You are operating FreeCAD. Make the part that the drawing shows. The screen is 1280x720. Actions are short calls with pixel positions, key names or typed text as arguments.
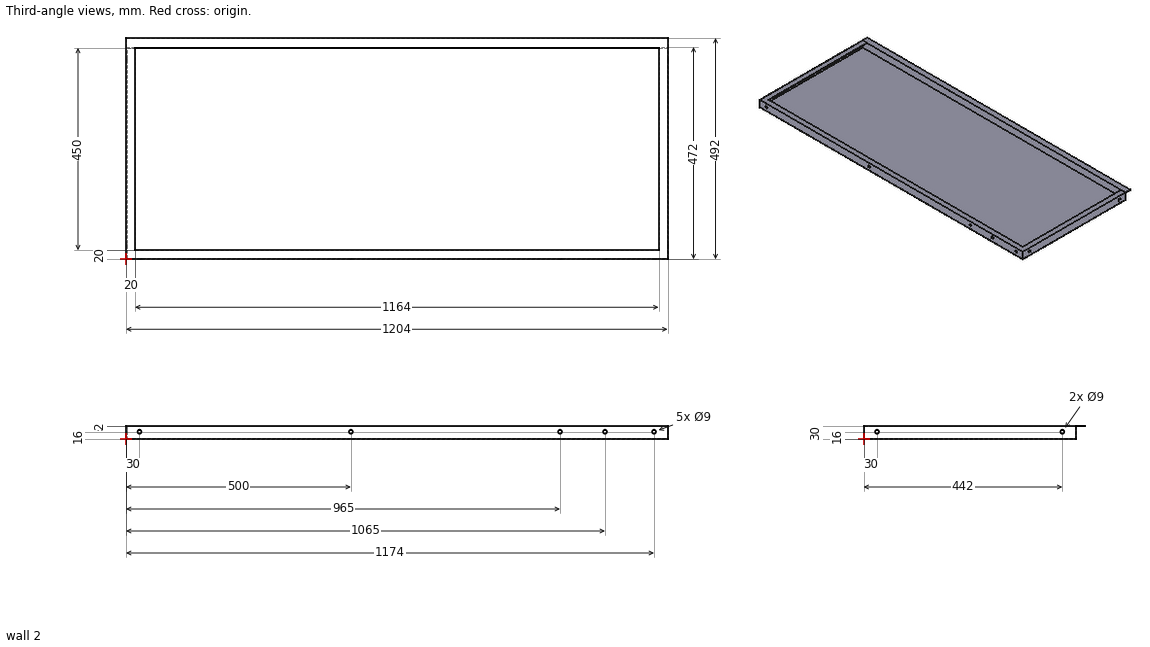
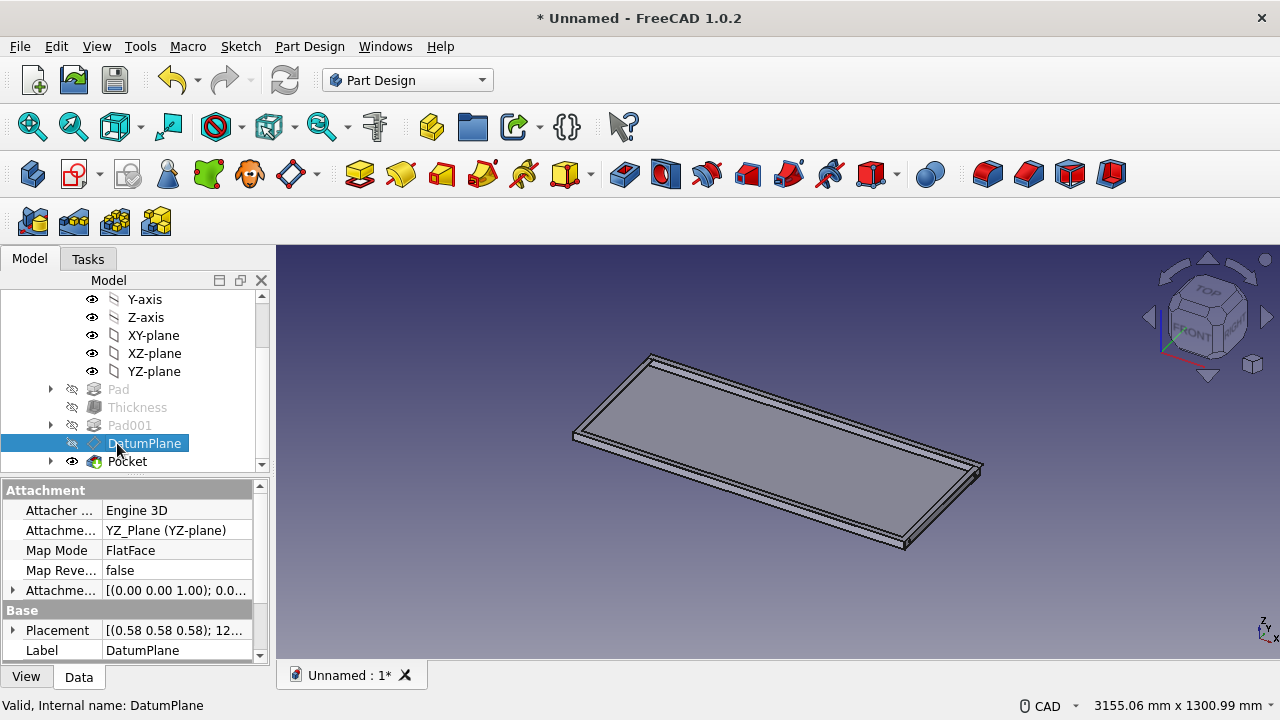
scroll(161, 385, down, 3)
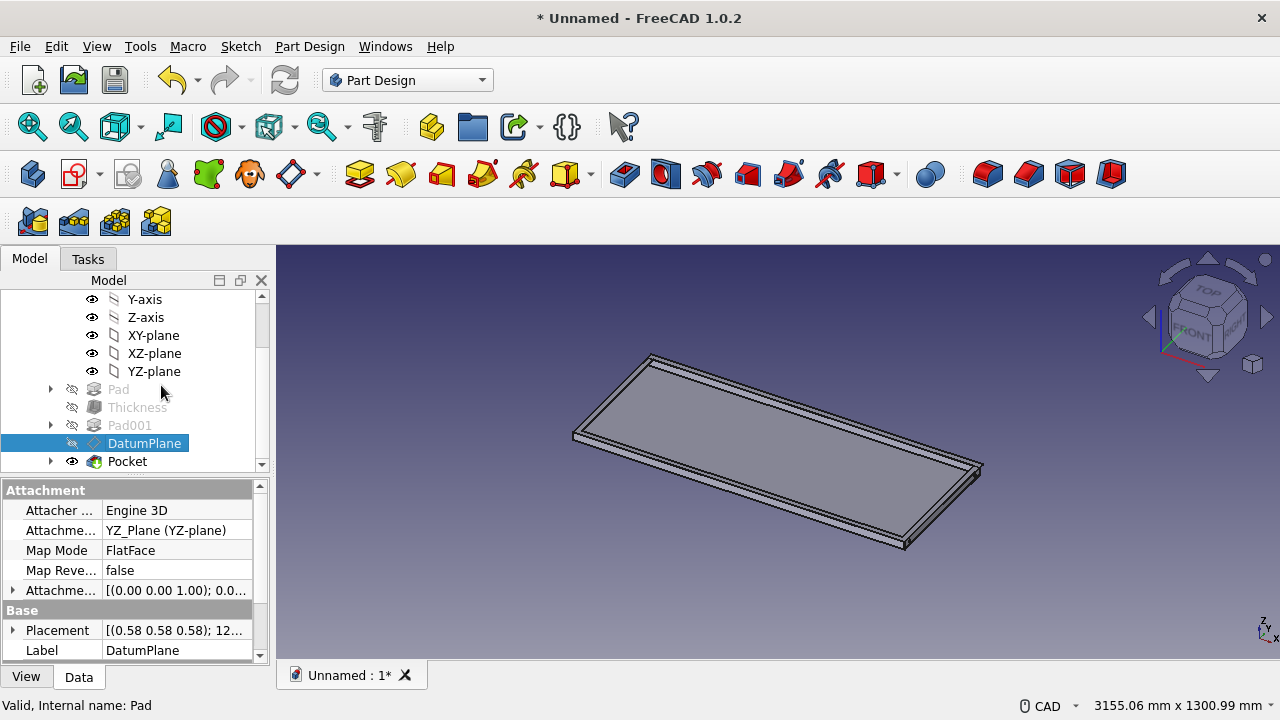
scroll(161, 385, up, 15)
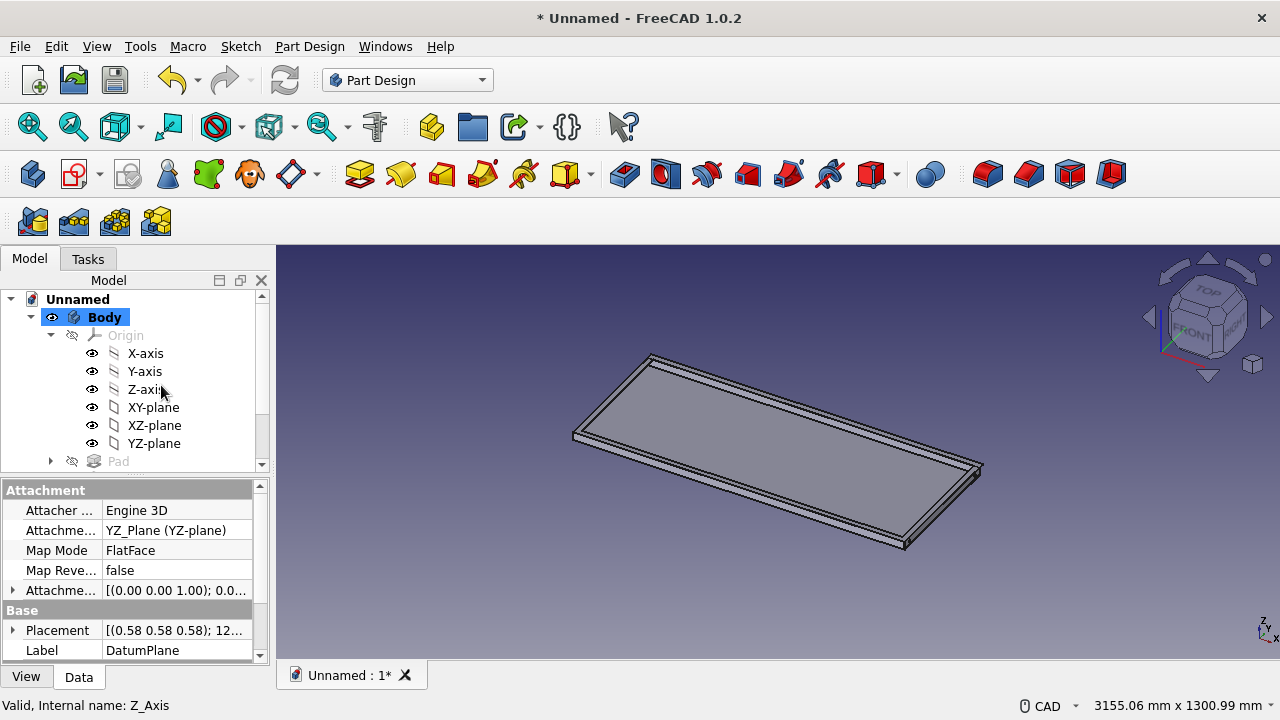
click(137, 425)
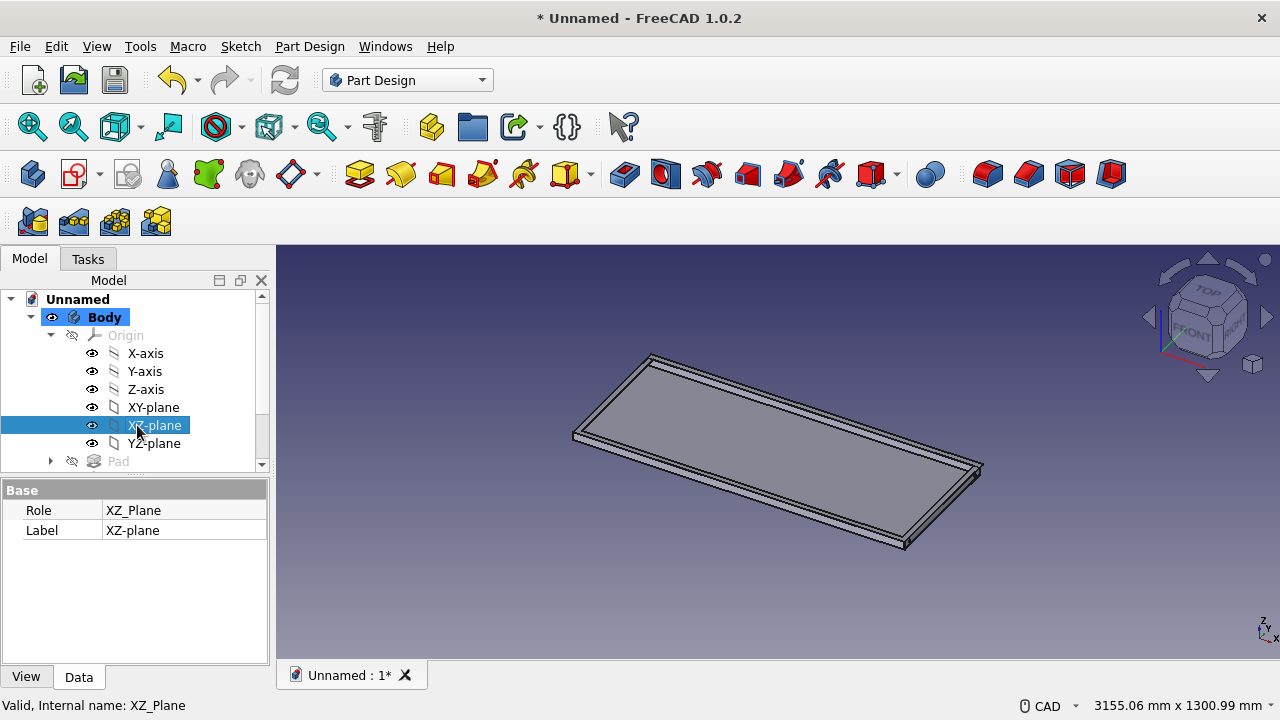
click(290, 174)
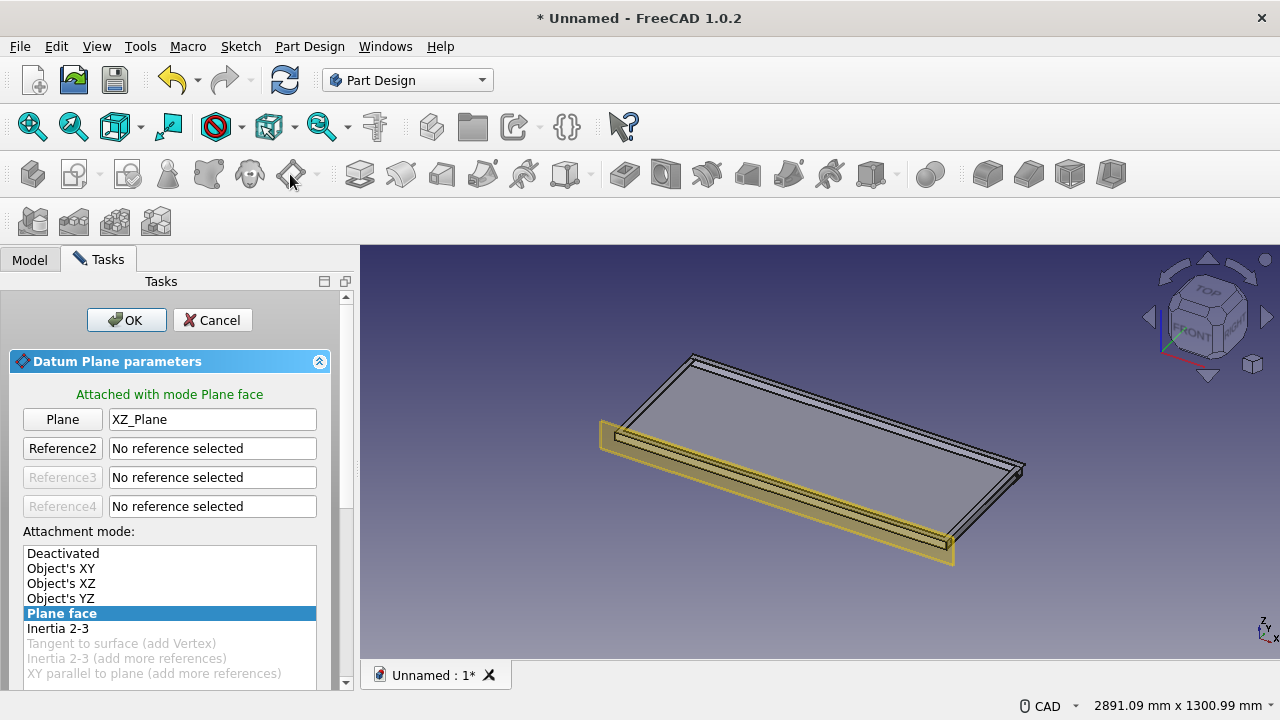
scroll(346, 490, down, 4)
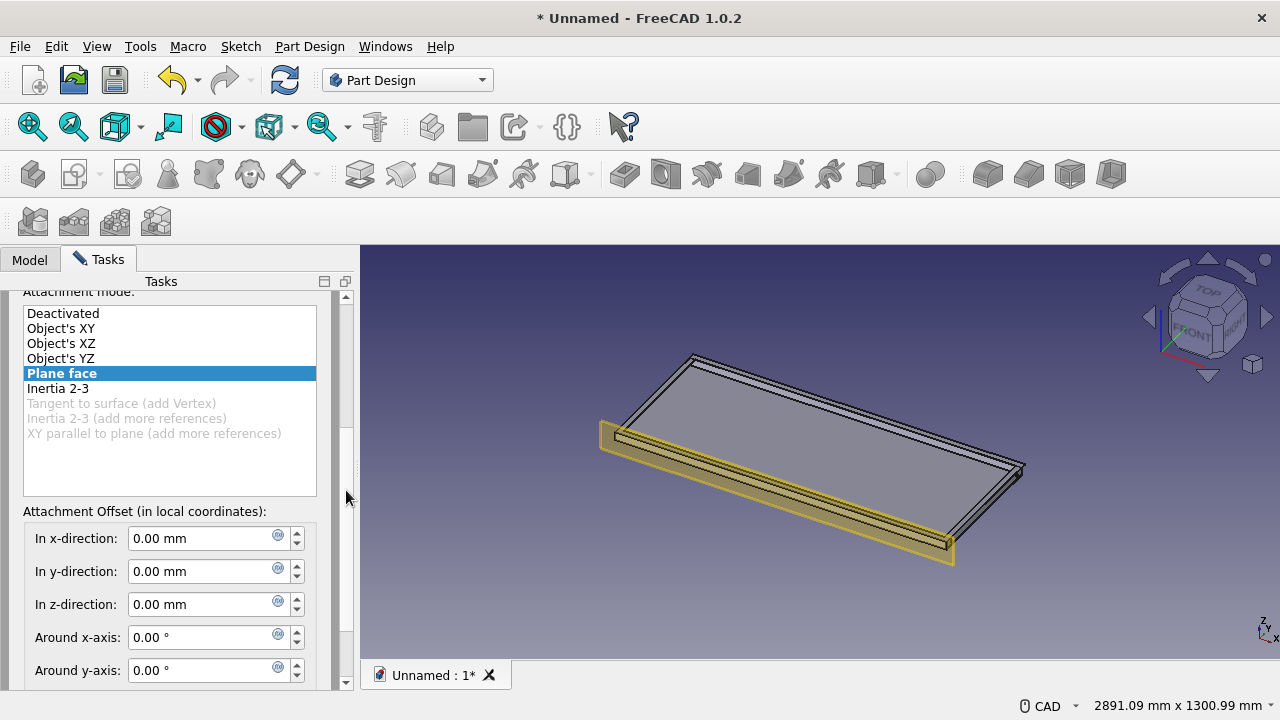
triple_click(210, 604)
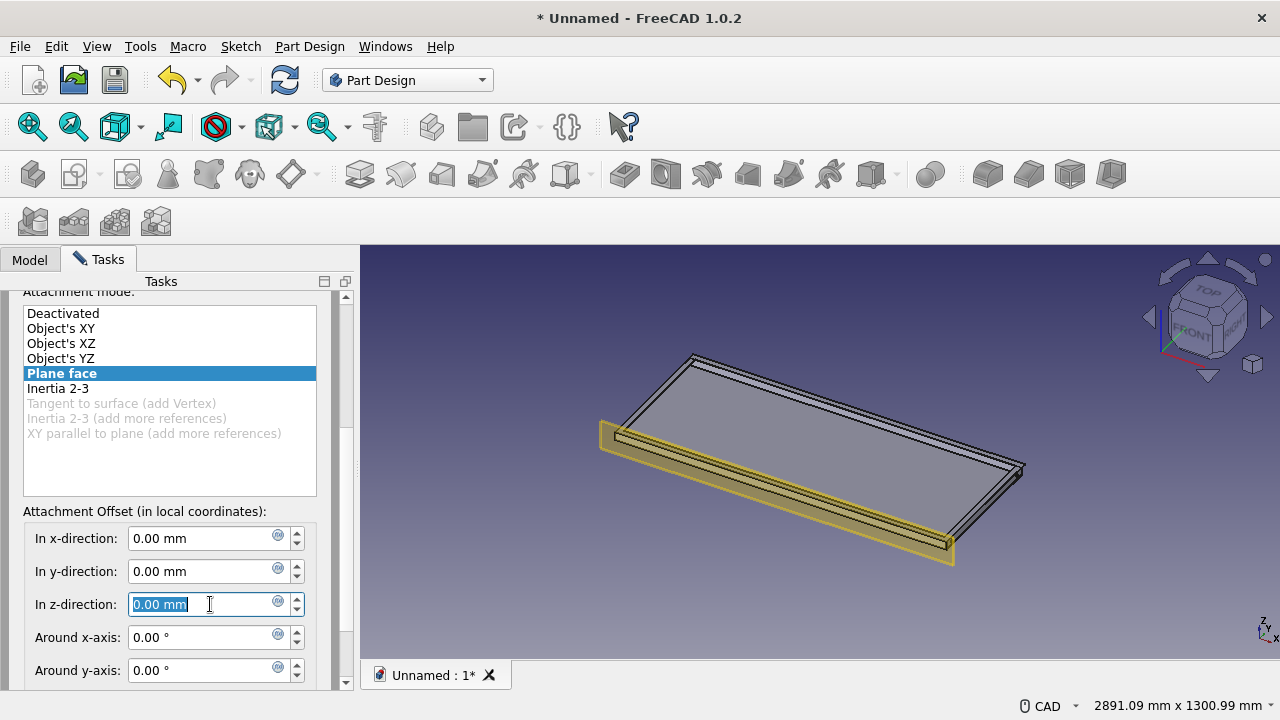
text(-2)
key(Tab)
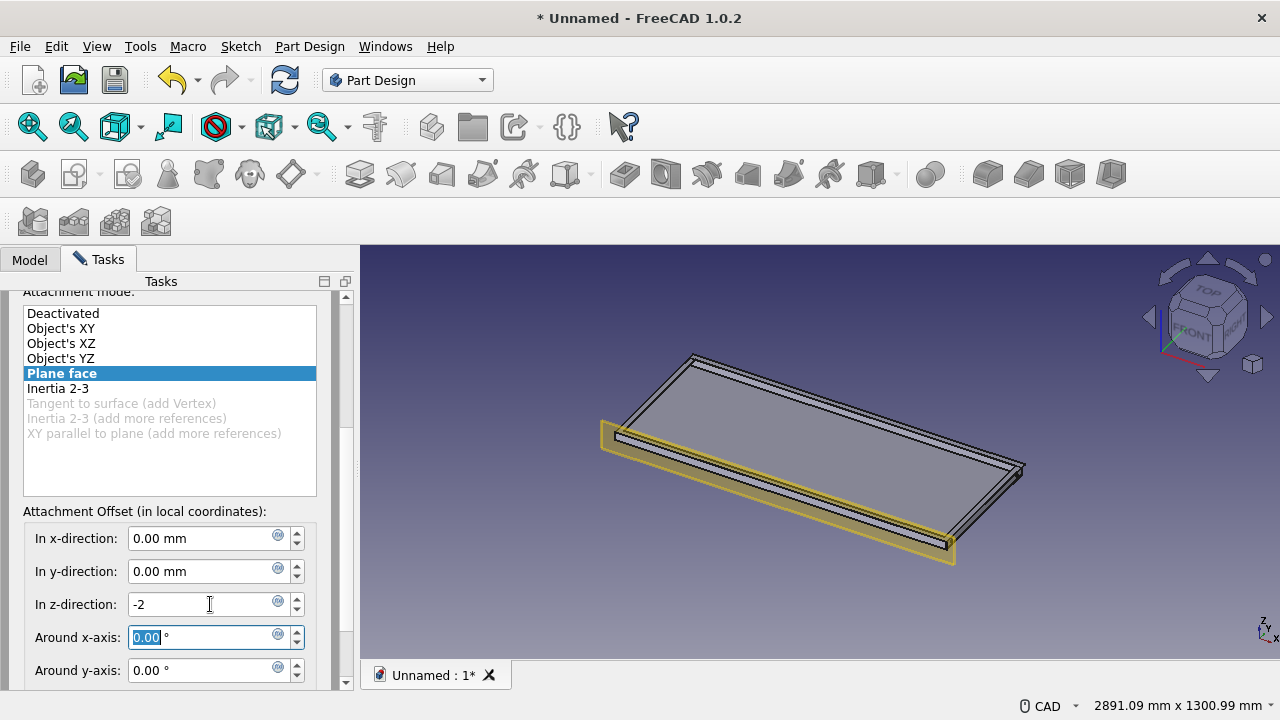
scroll(346, 490, up, 5)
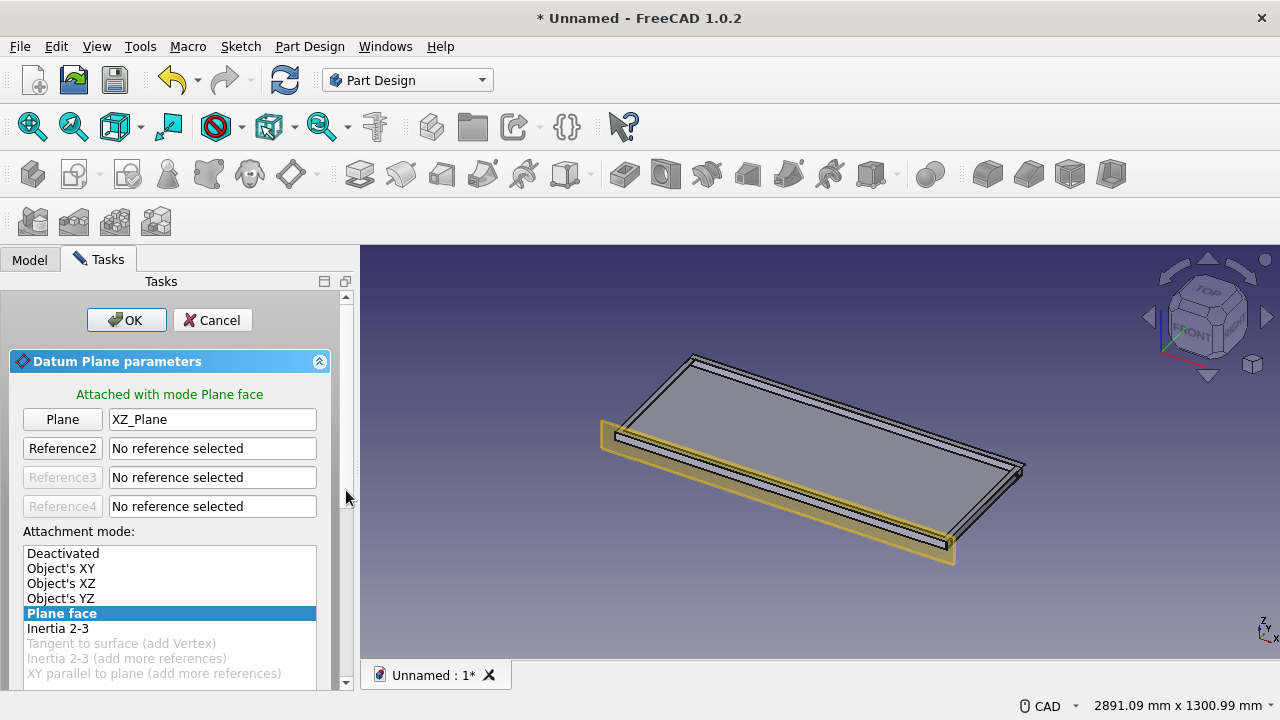
click(127, 320)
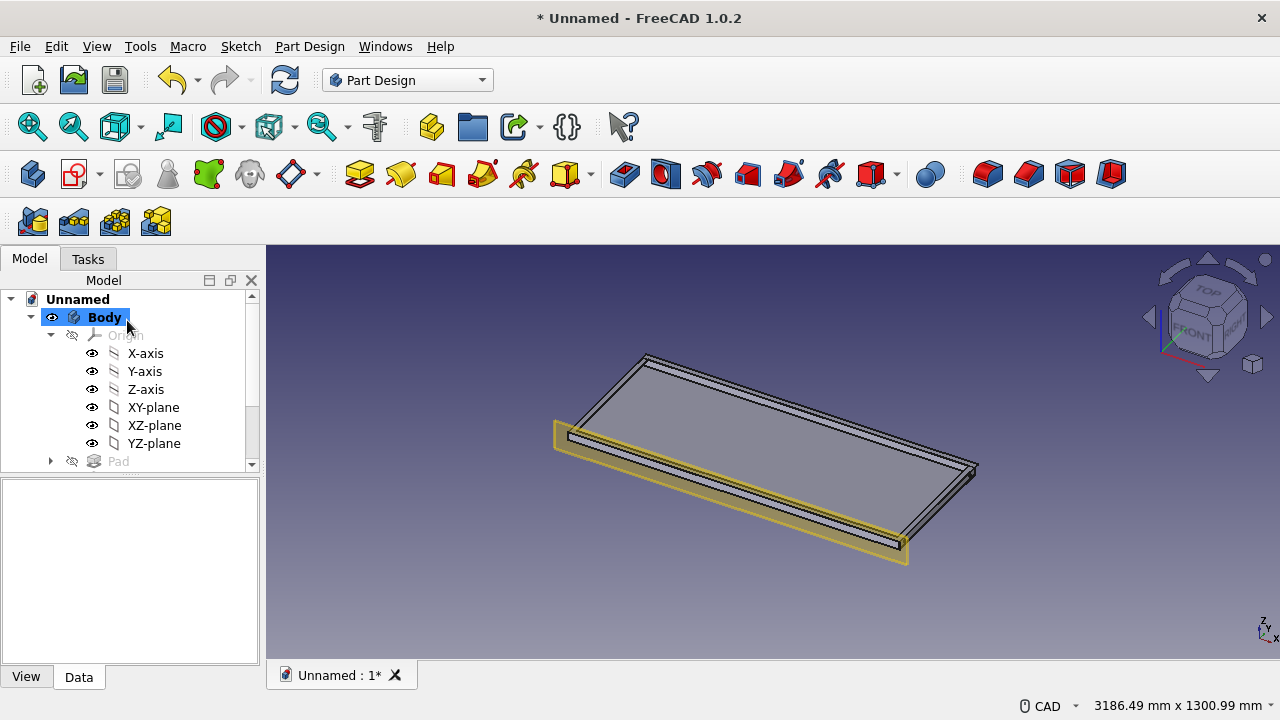
scroll(101, 385, down, 3)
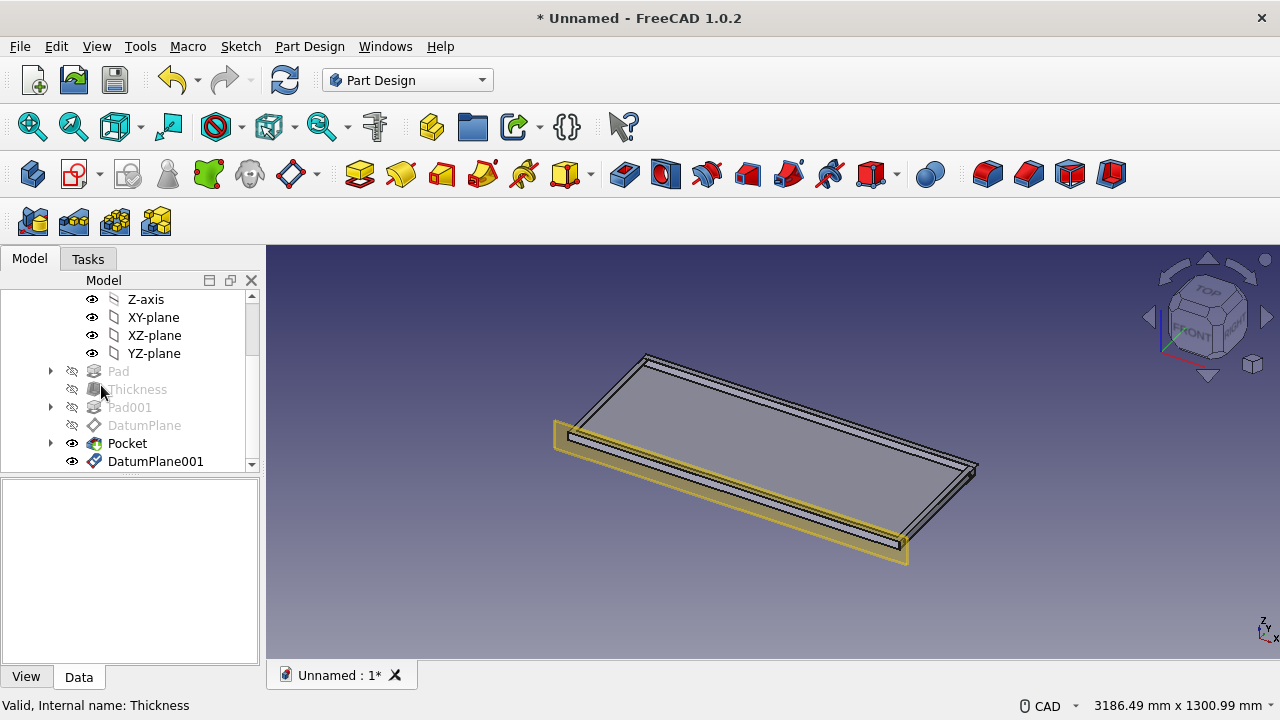
click(117, 461)